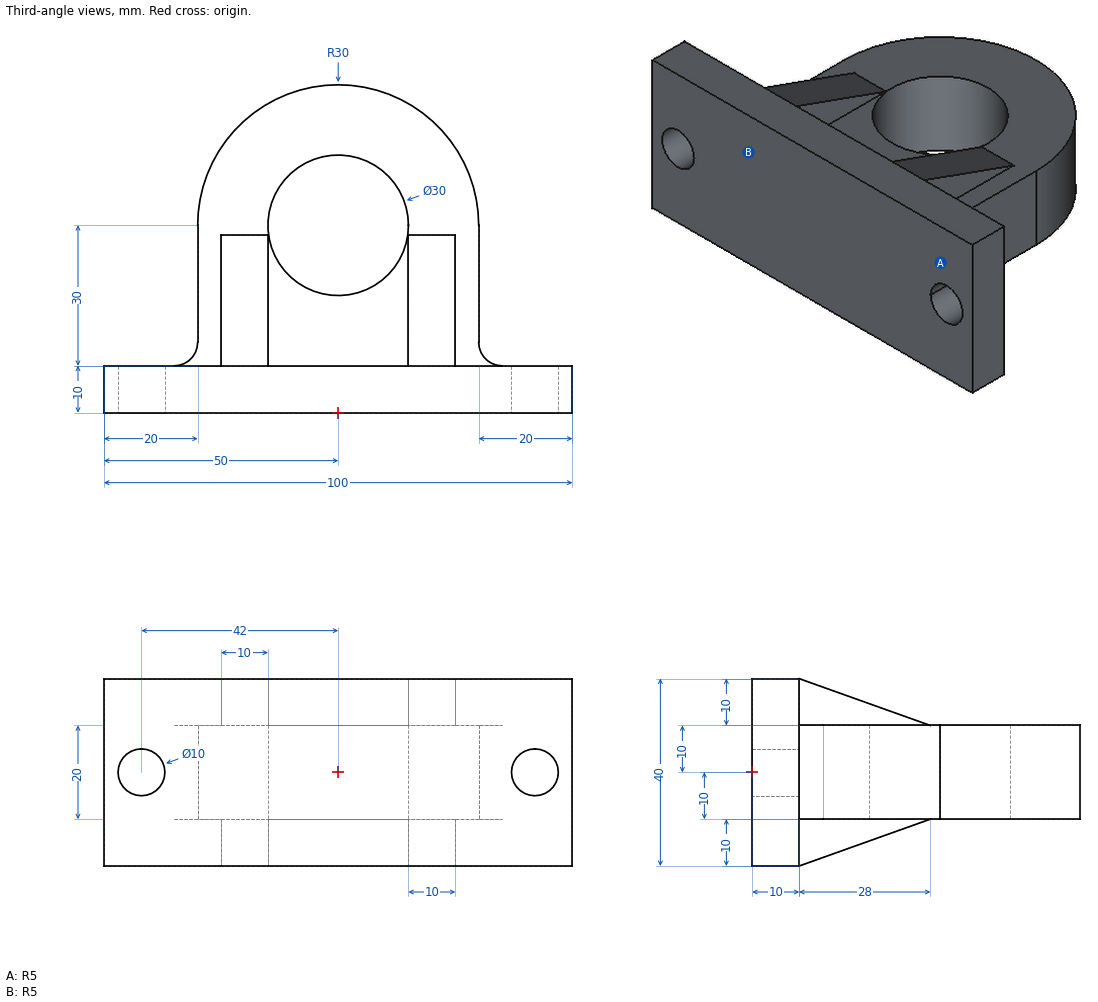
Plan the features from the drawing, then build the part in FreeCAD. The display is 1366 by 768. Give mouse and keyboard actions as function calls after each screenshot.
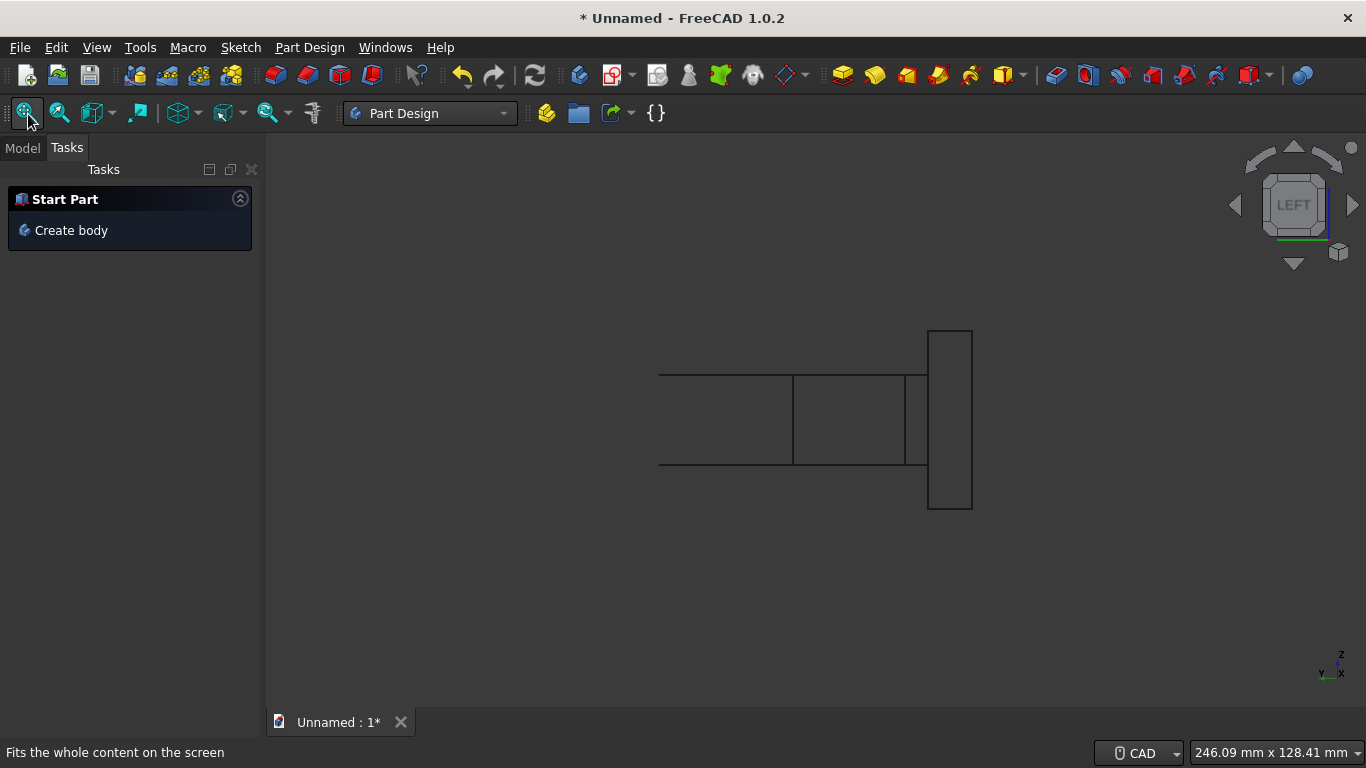
key(0)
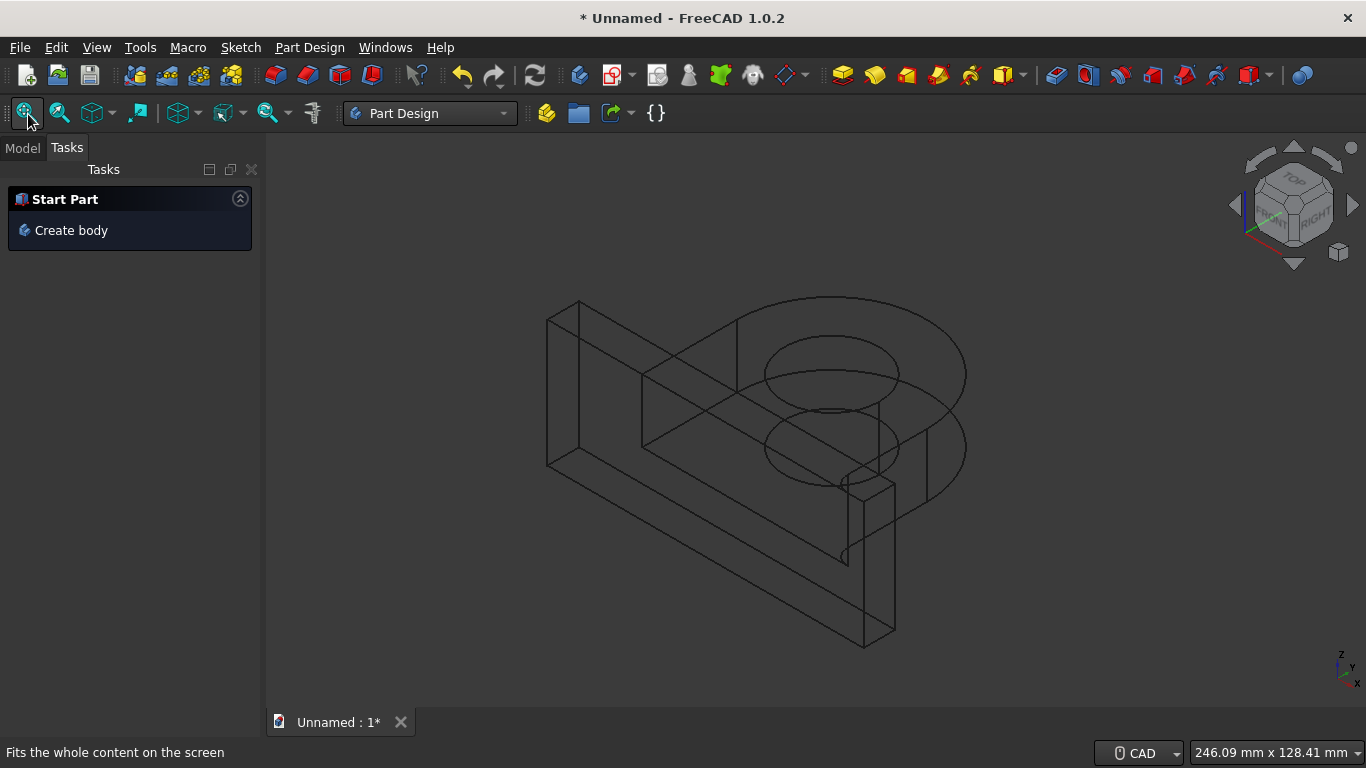
click(642, 410)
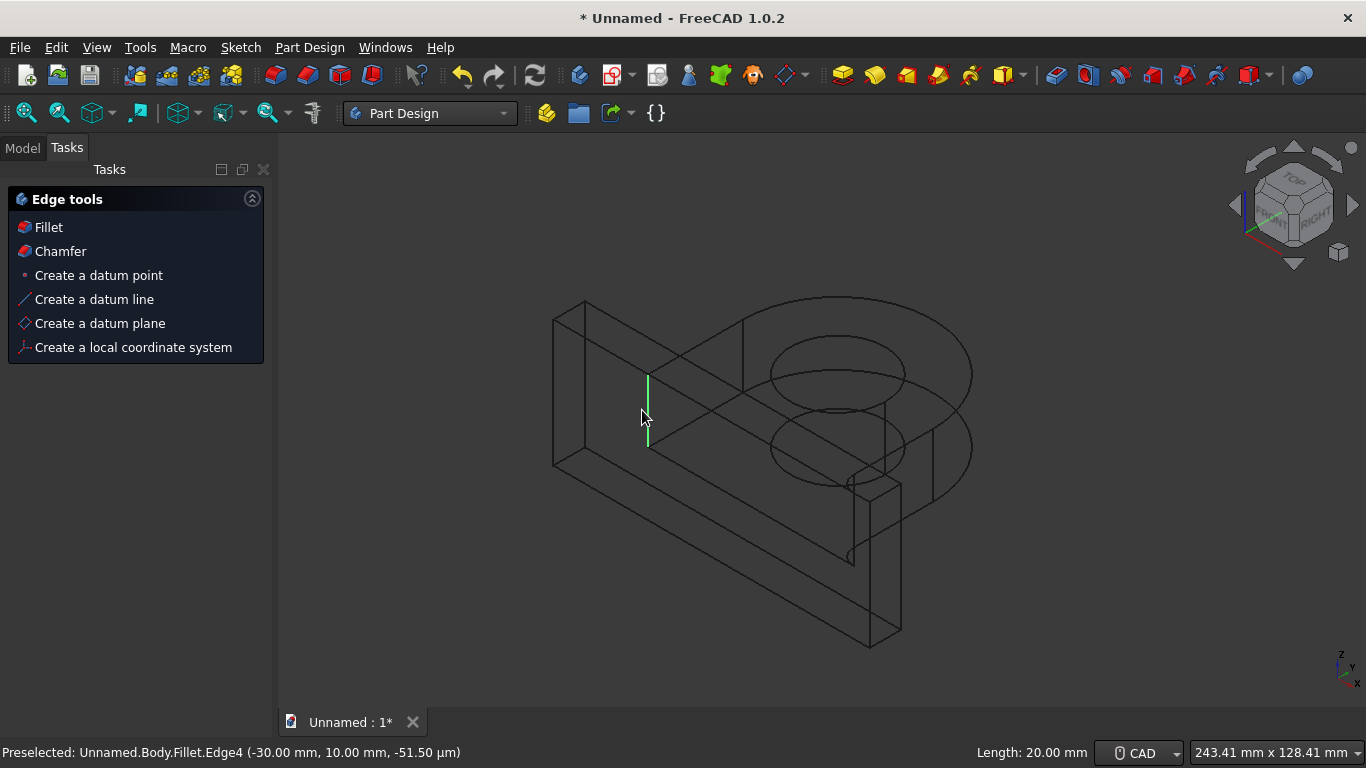
key(v)
key(1)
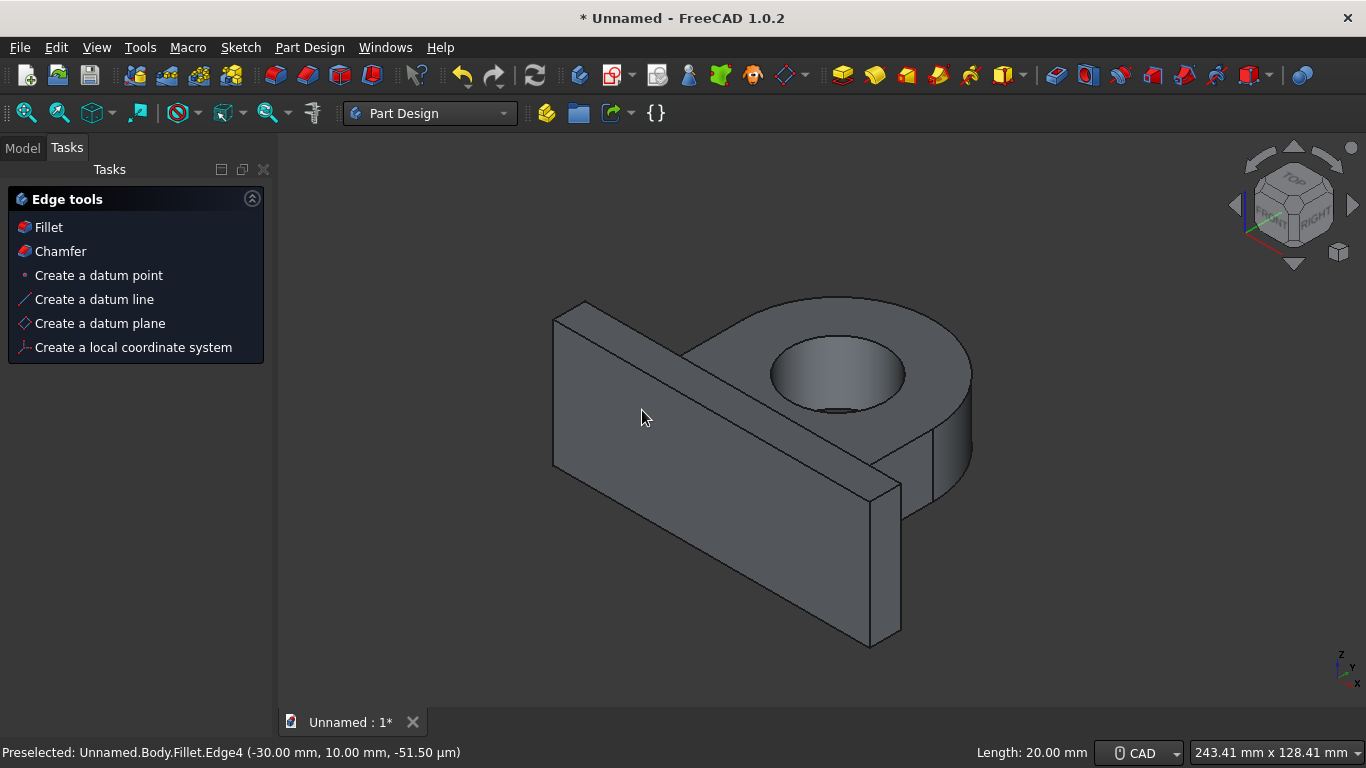
click(276, 76)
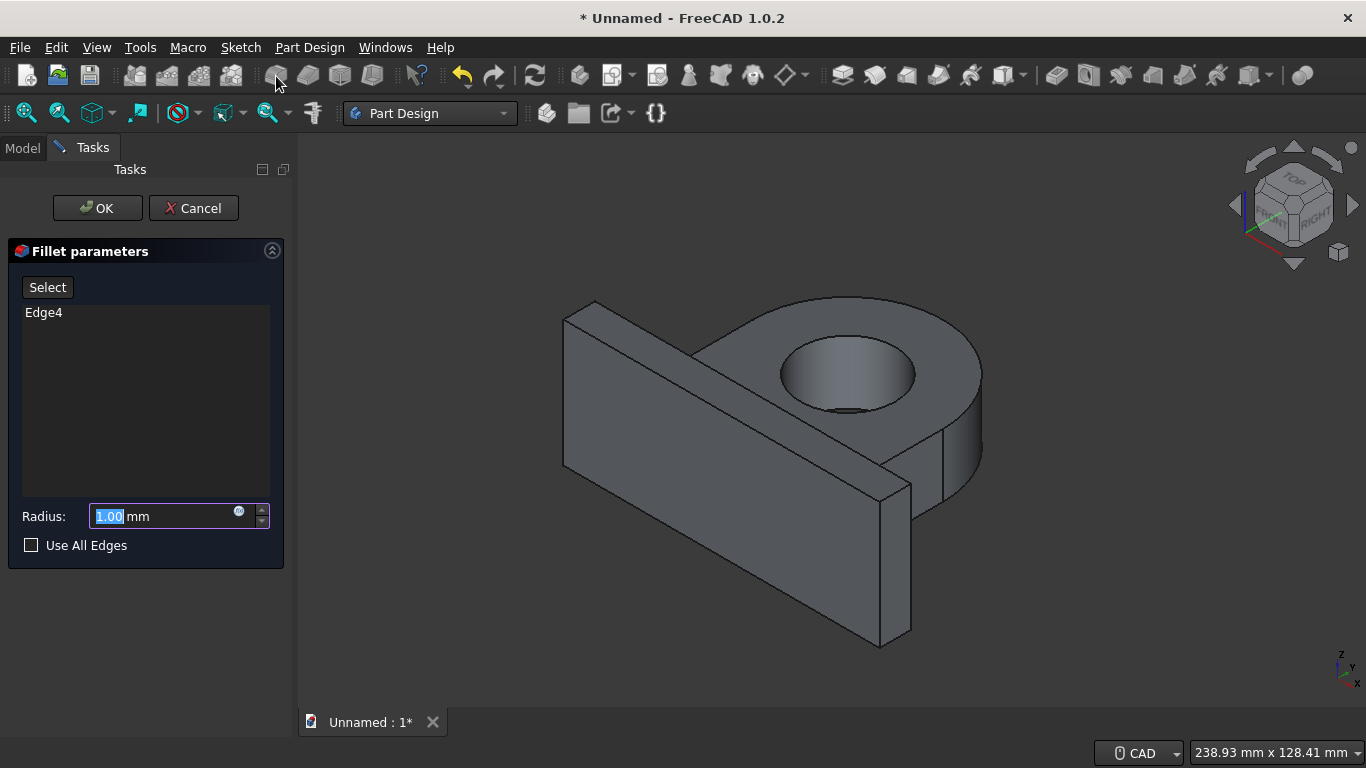
text(5)
key(Tab)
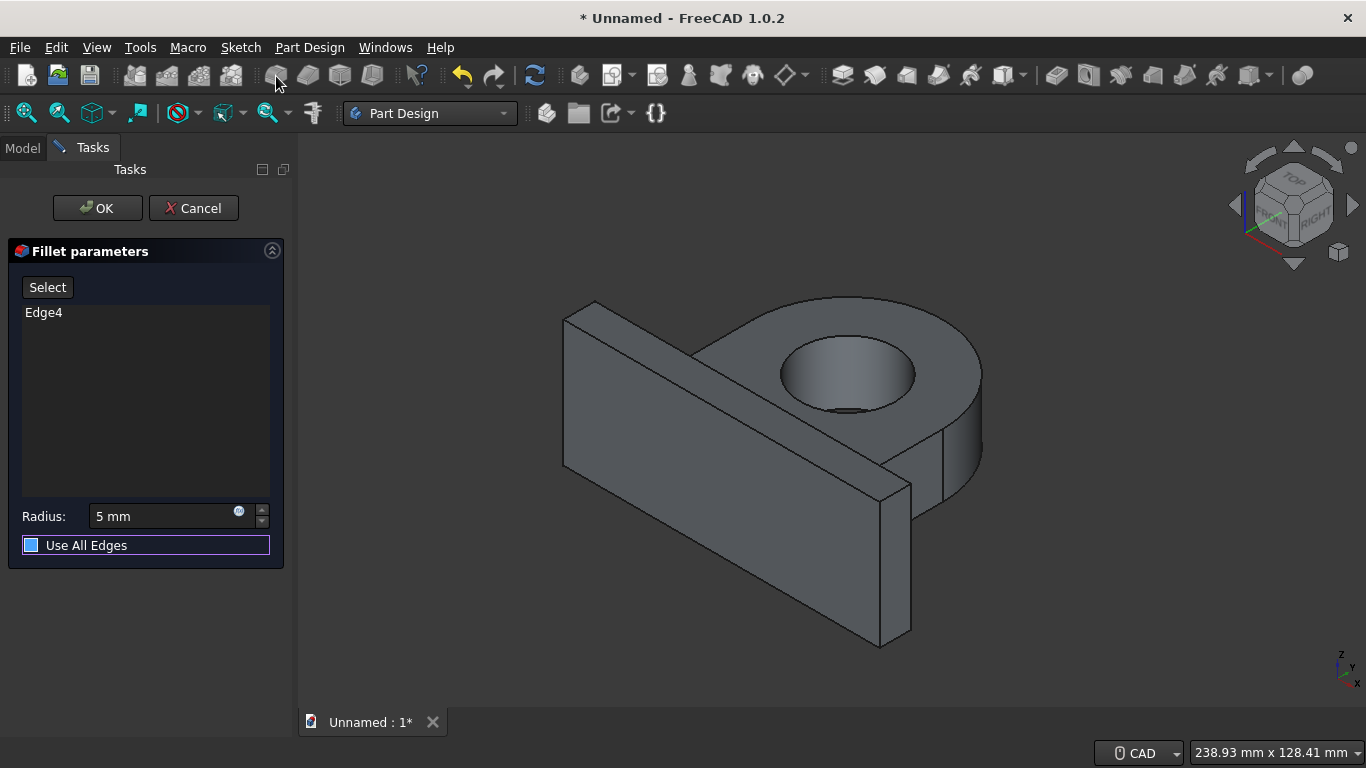
click(98, 208)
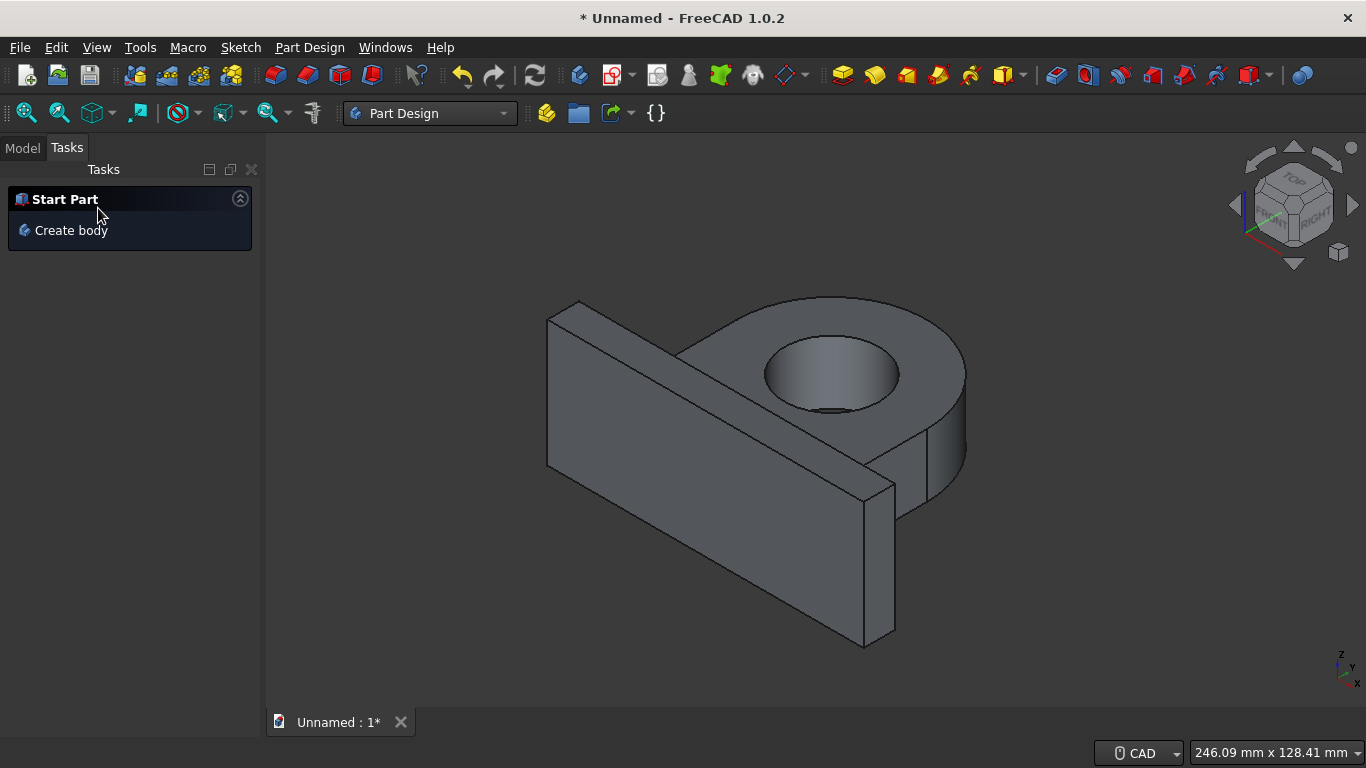
click(23, 147)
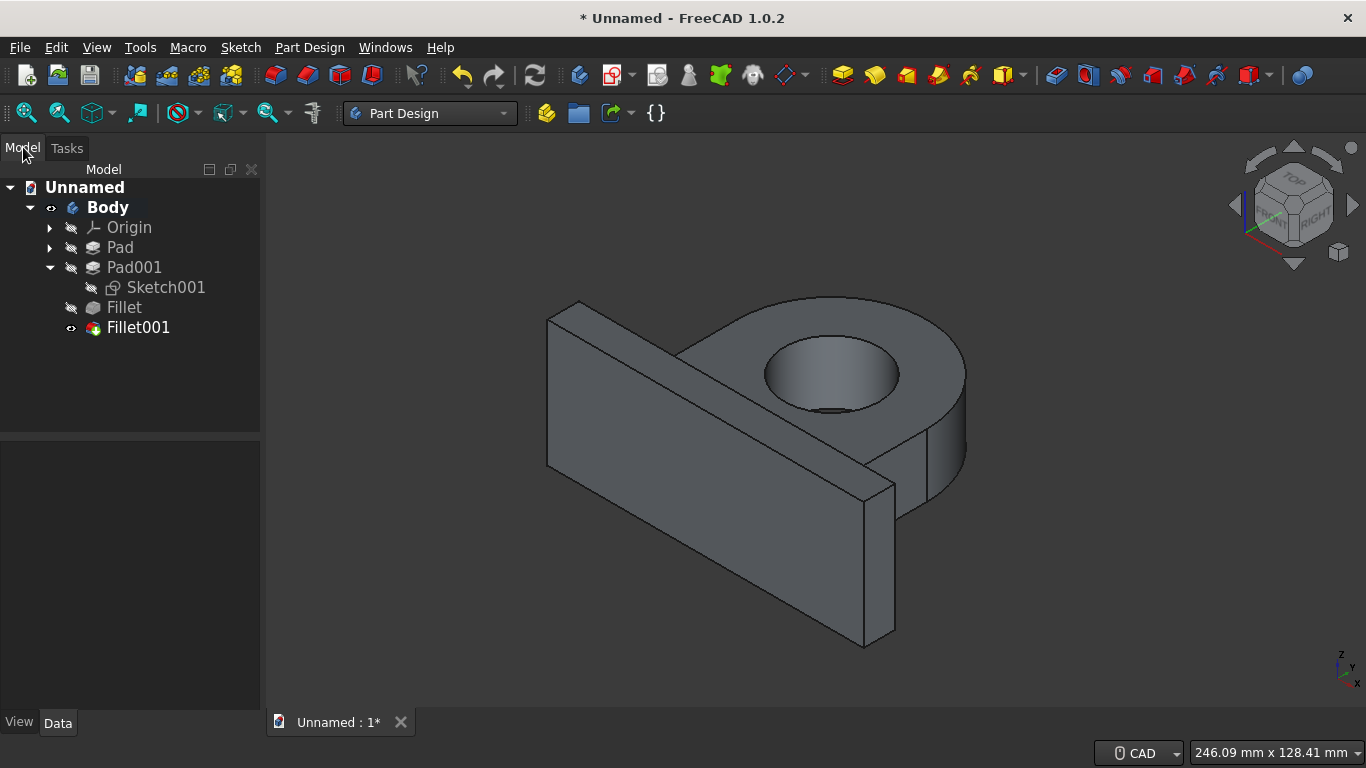
click(50, 228)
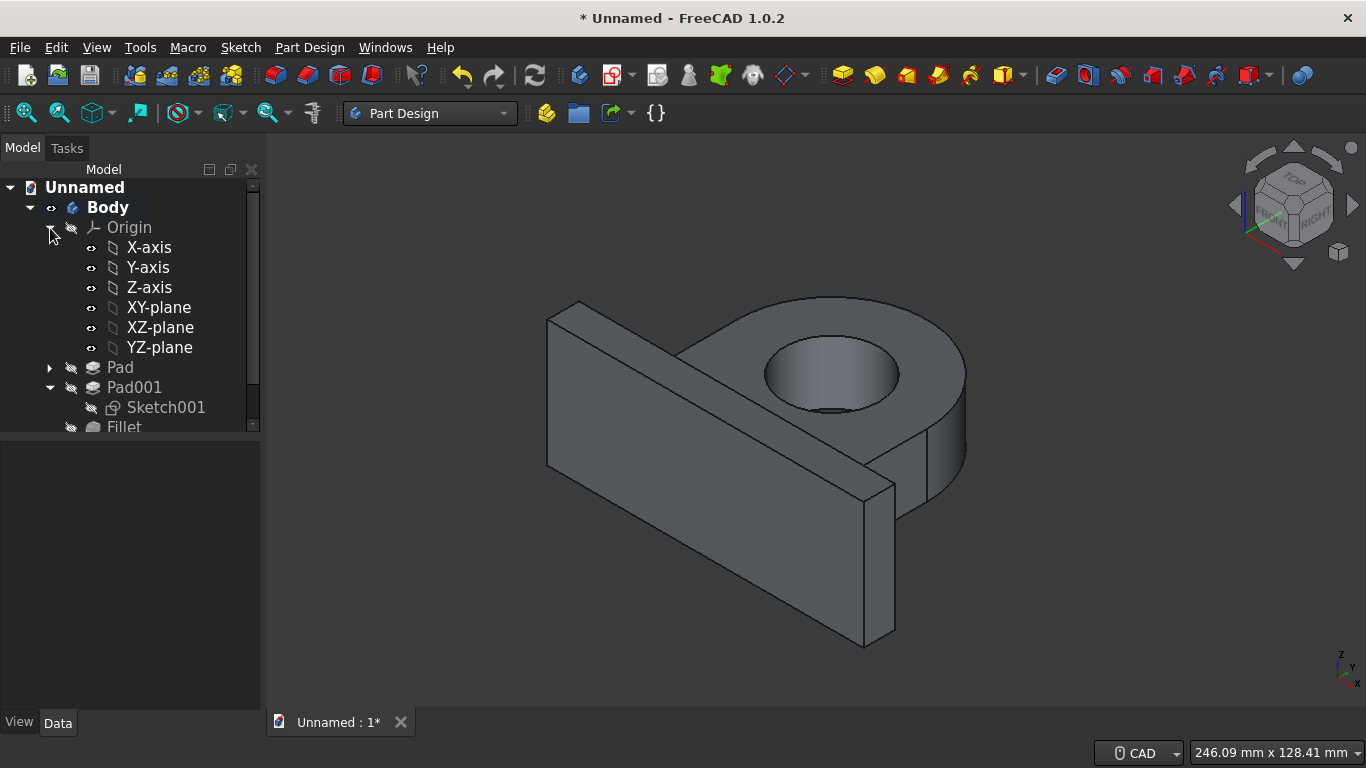
click(136, 348)